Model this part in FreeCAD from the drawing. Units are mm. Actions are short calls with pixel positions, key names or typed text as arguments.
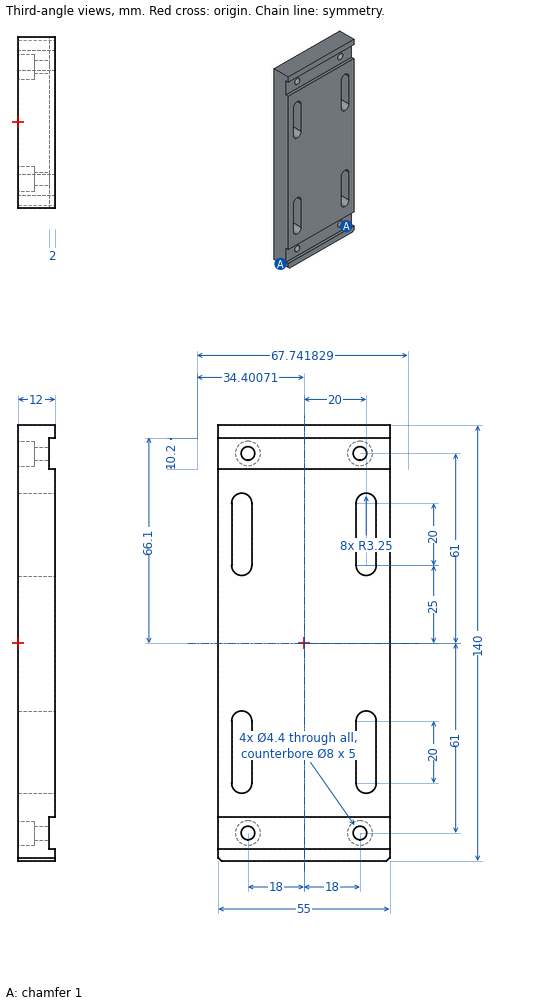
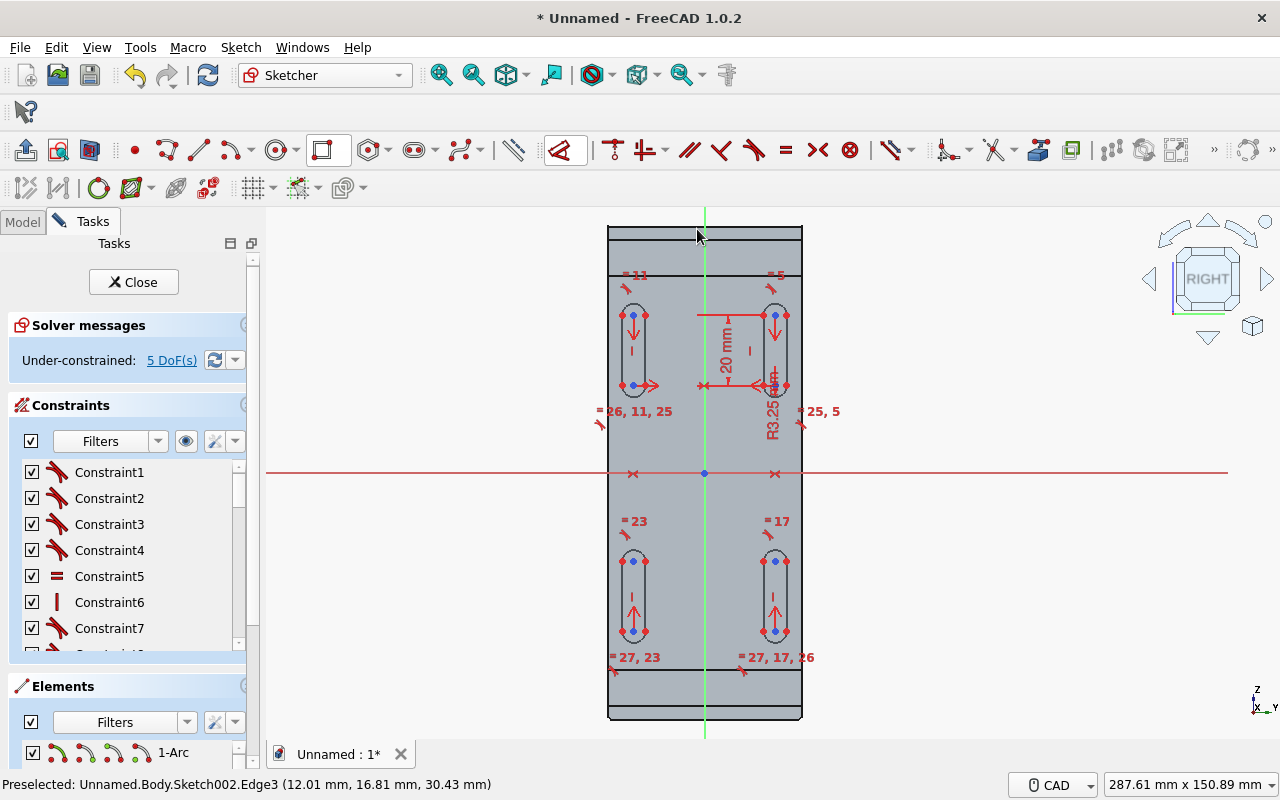
click(622, 365)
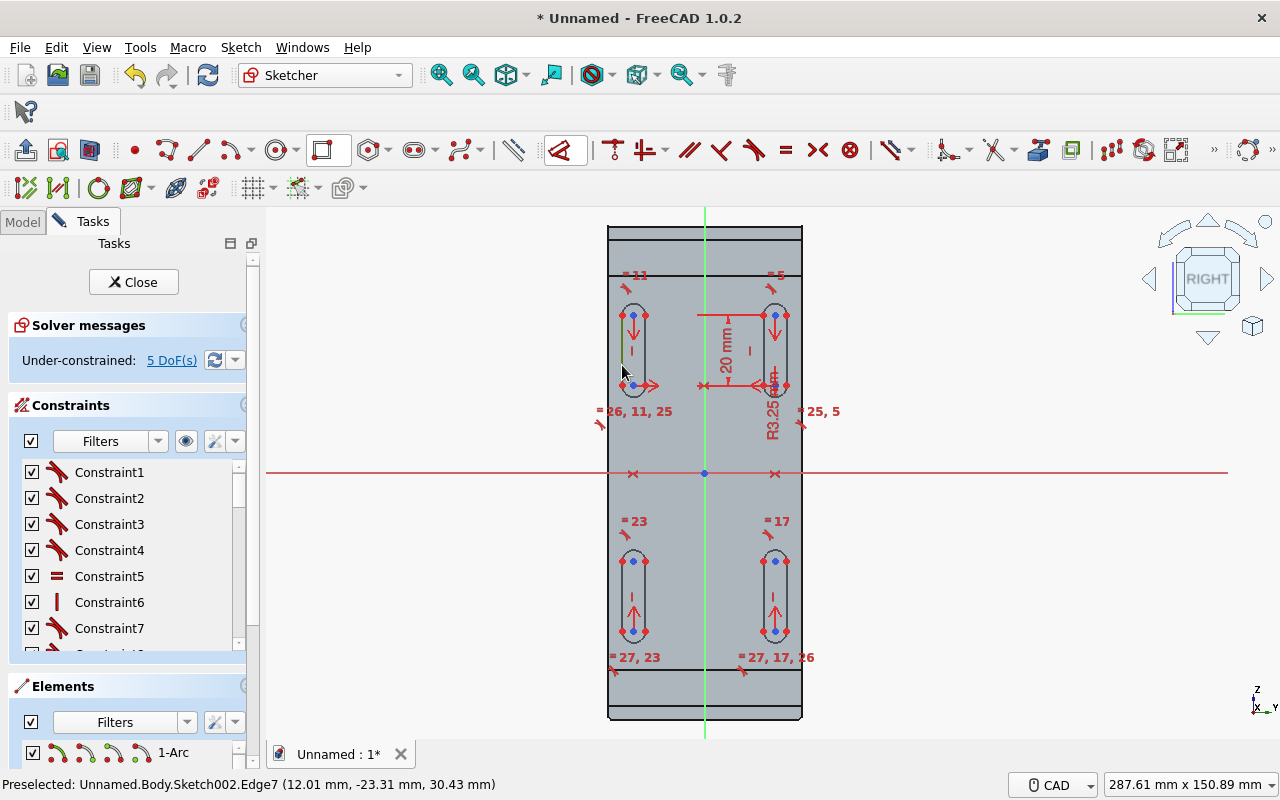
click(582, 150)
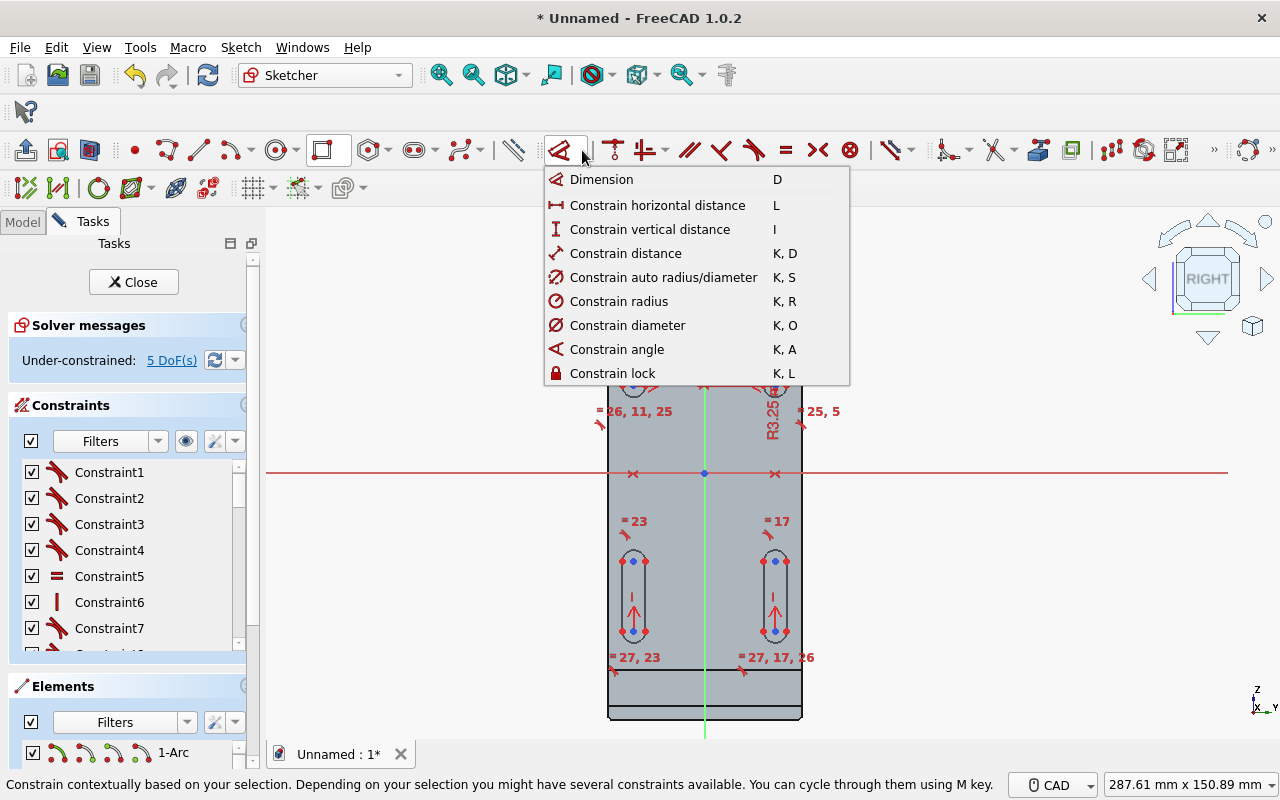
click(697, 229)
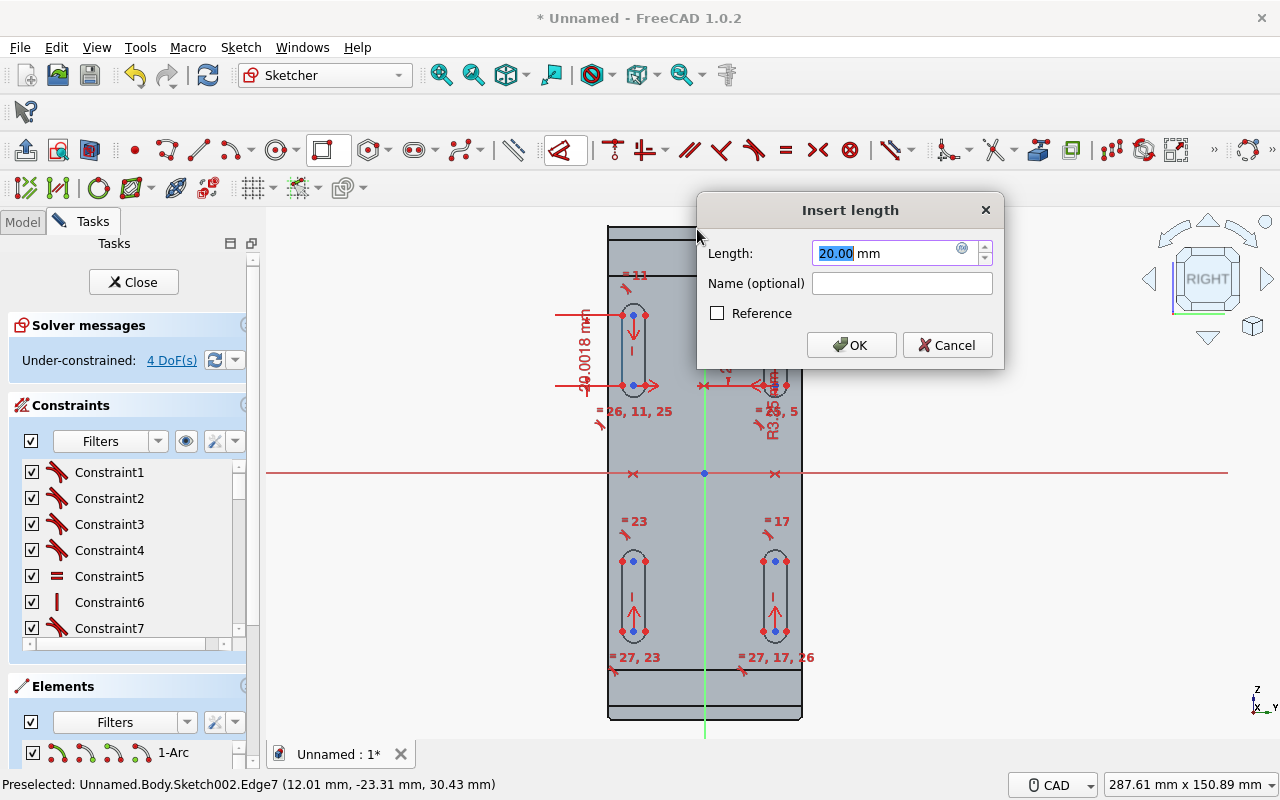
text(20)
key(Return)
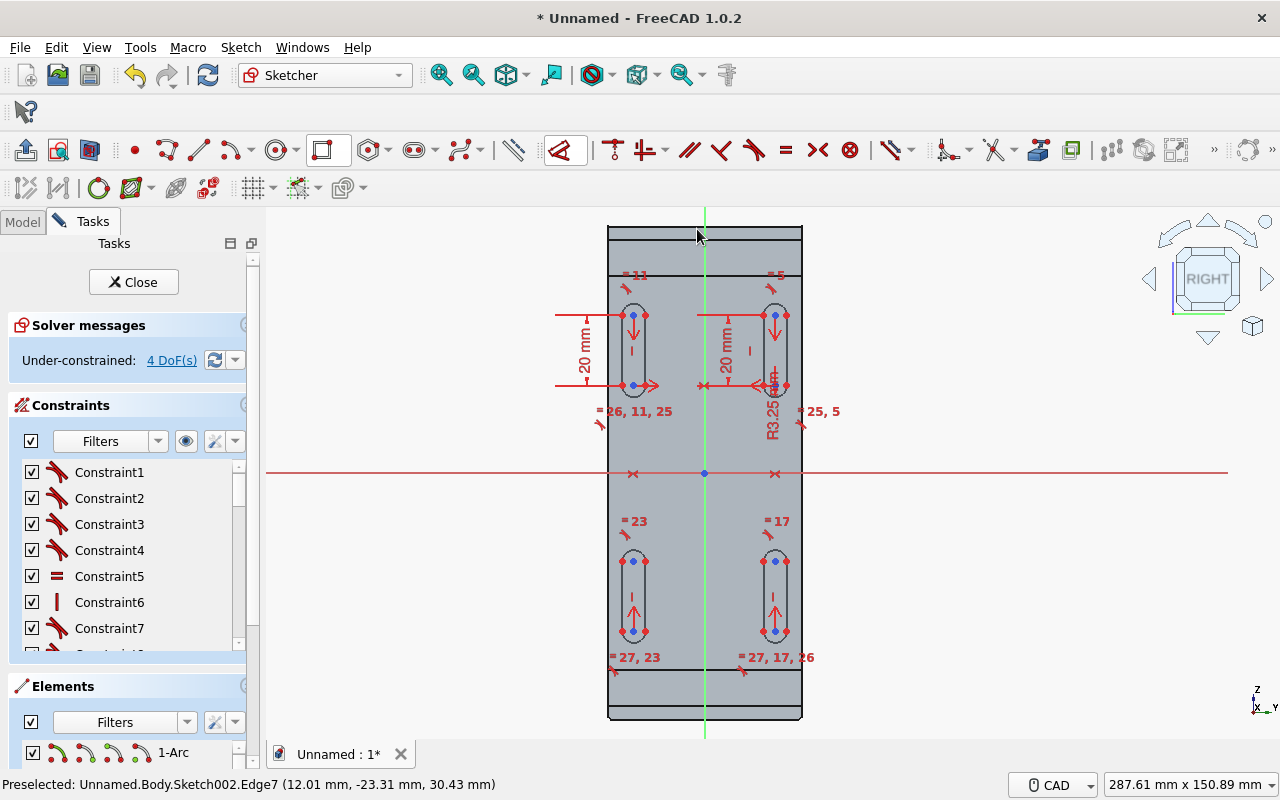
click(764, 610)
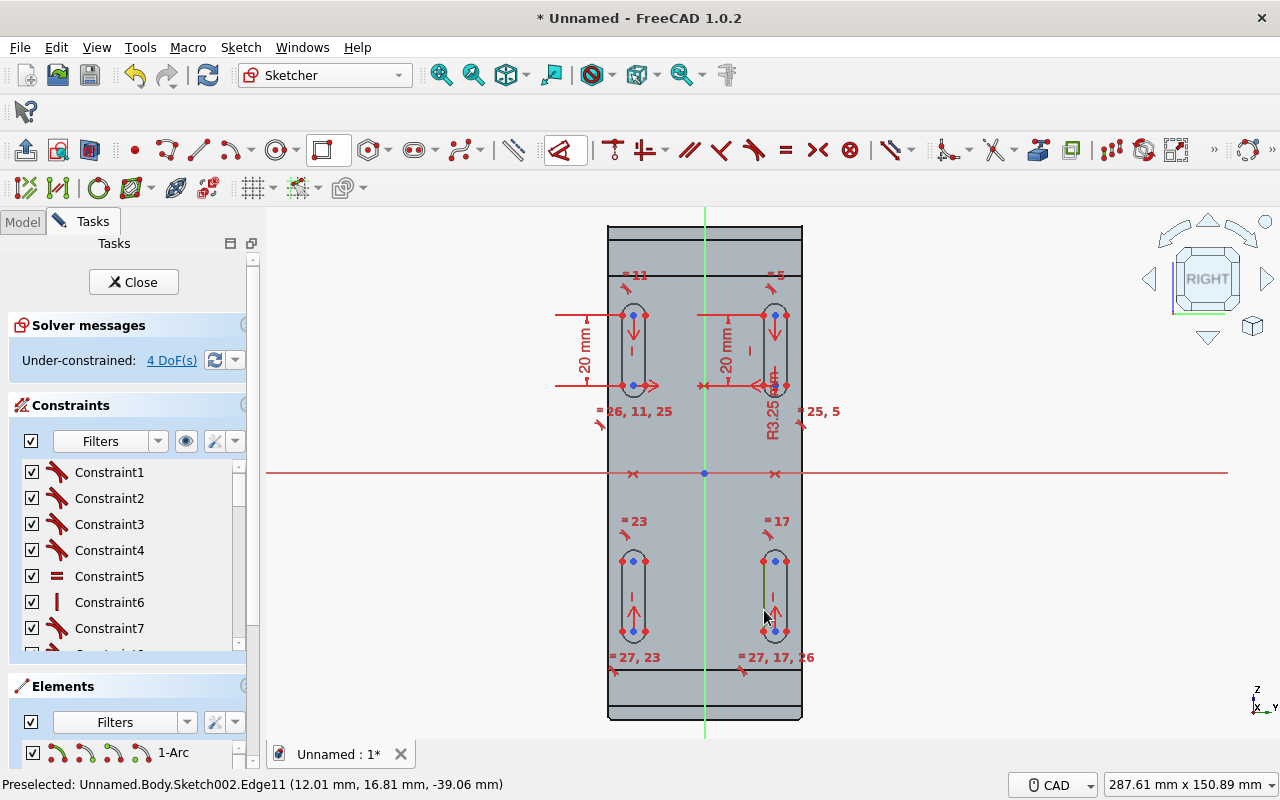
key(i)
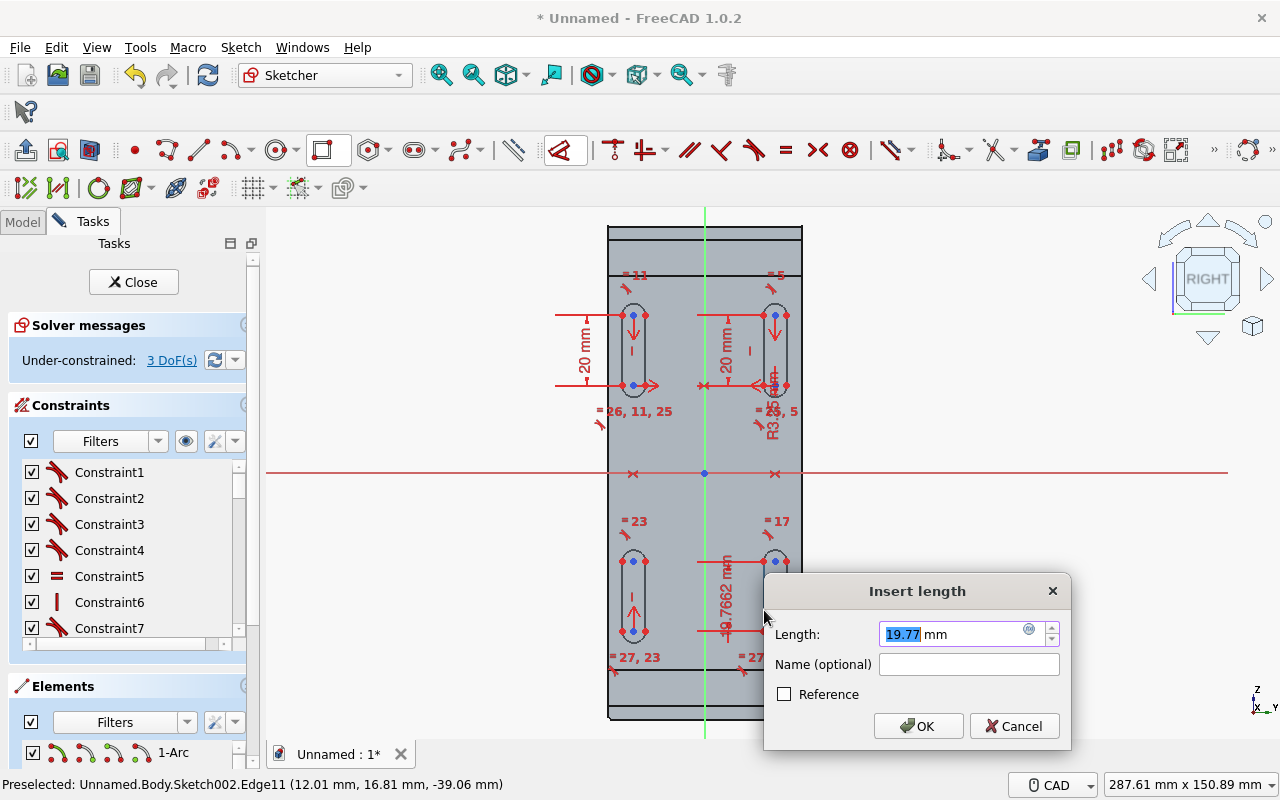
text(20)
key(Return)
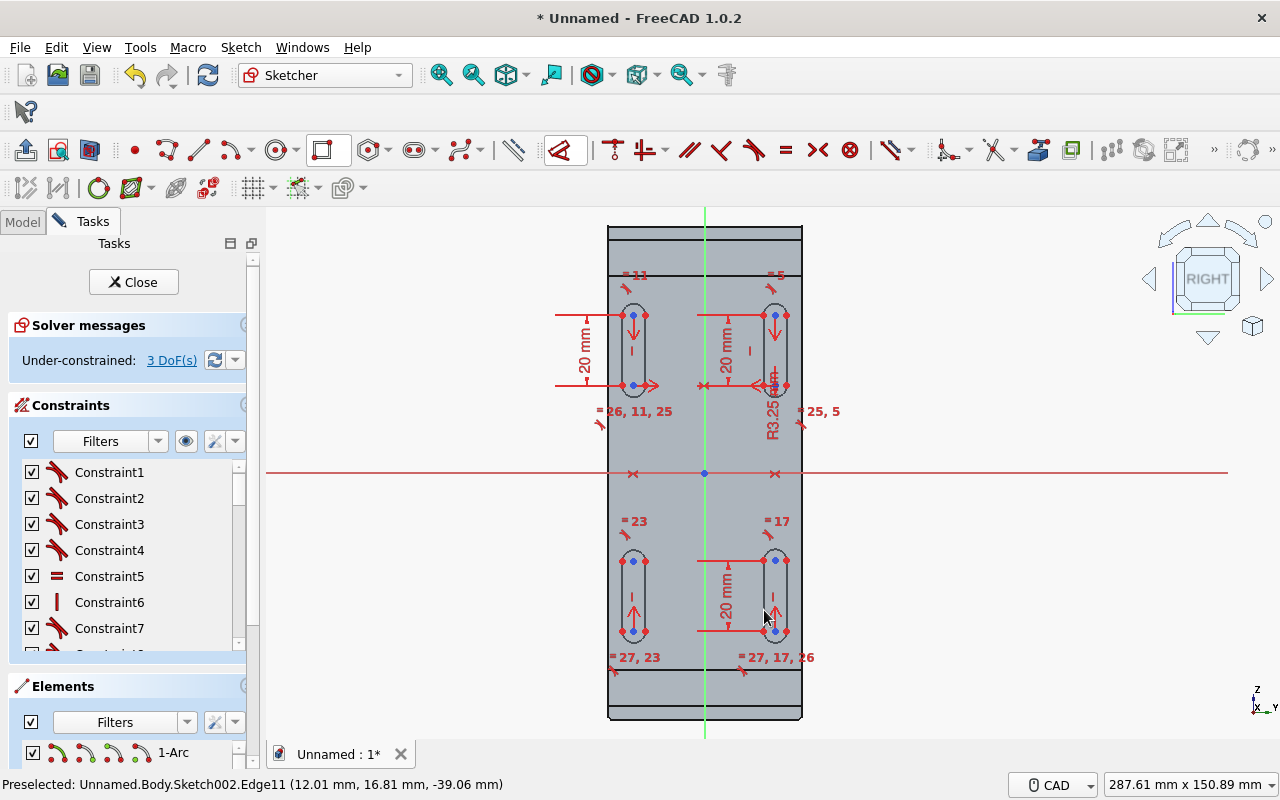
click(622, 610)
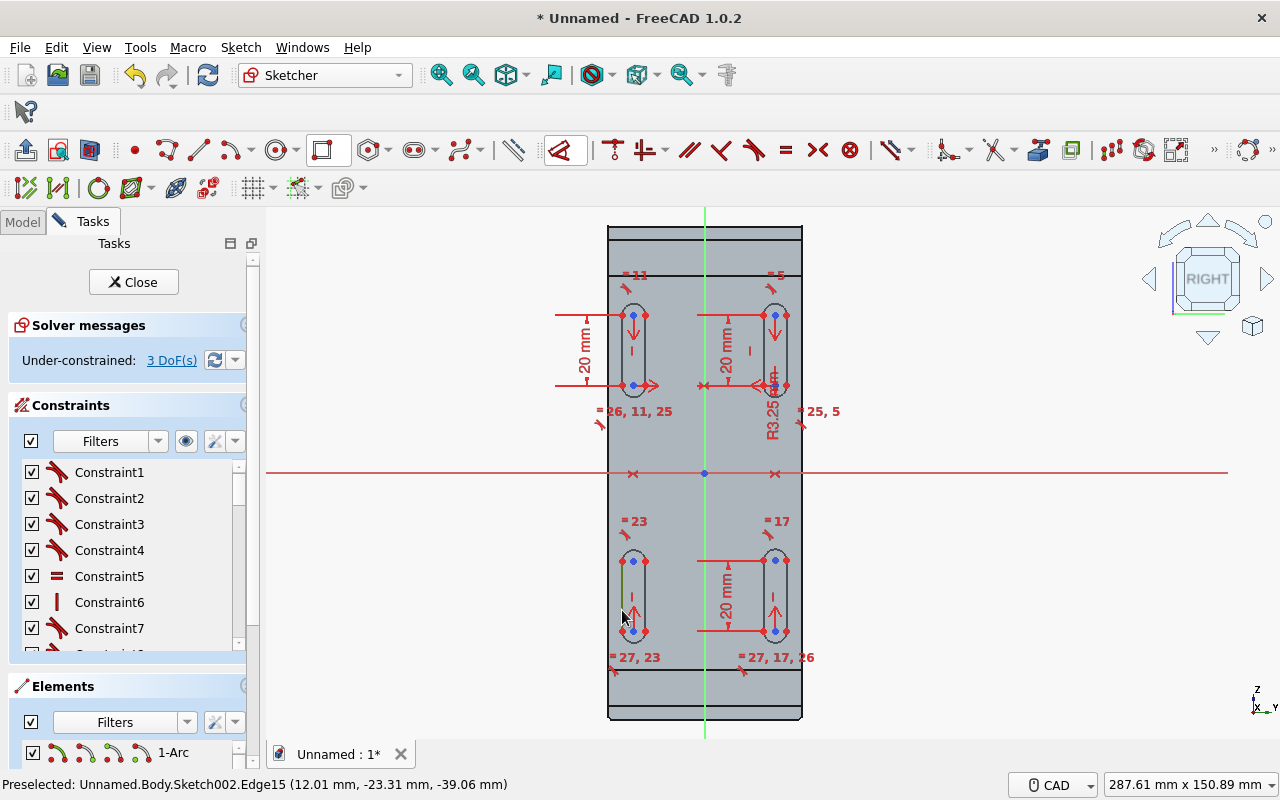
click(582, 150)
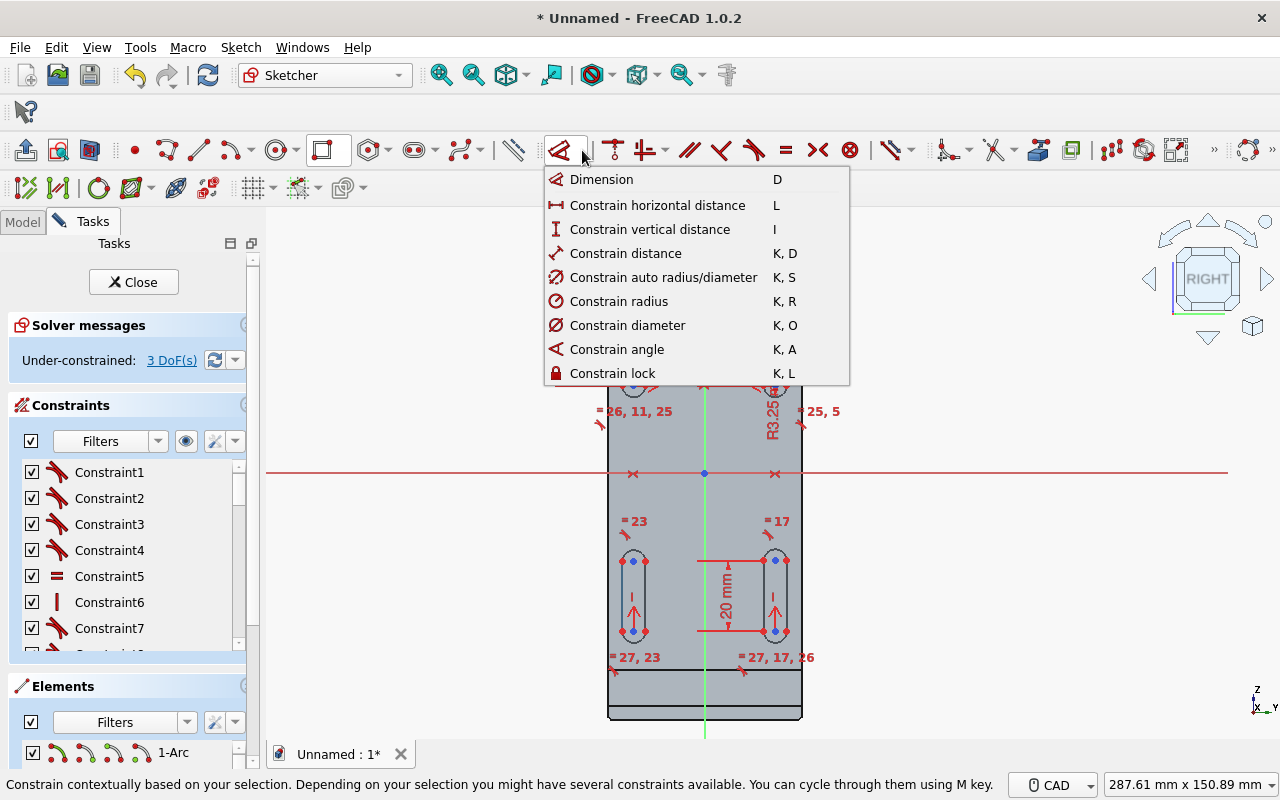
click(697, 229)